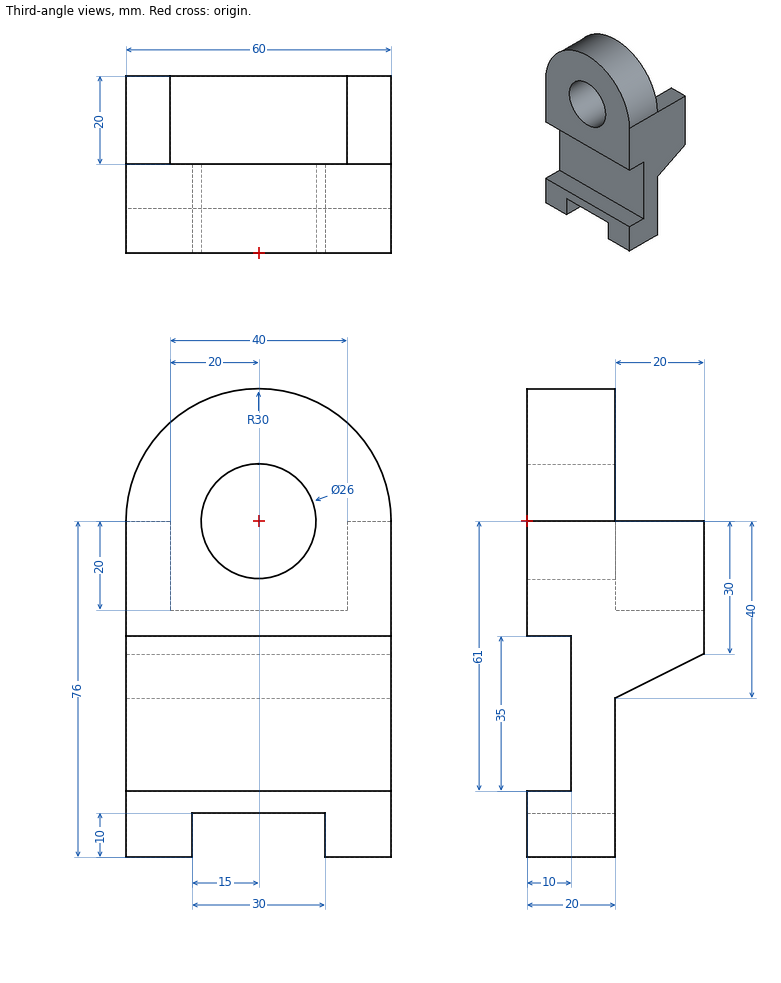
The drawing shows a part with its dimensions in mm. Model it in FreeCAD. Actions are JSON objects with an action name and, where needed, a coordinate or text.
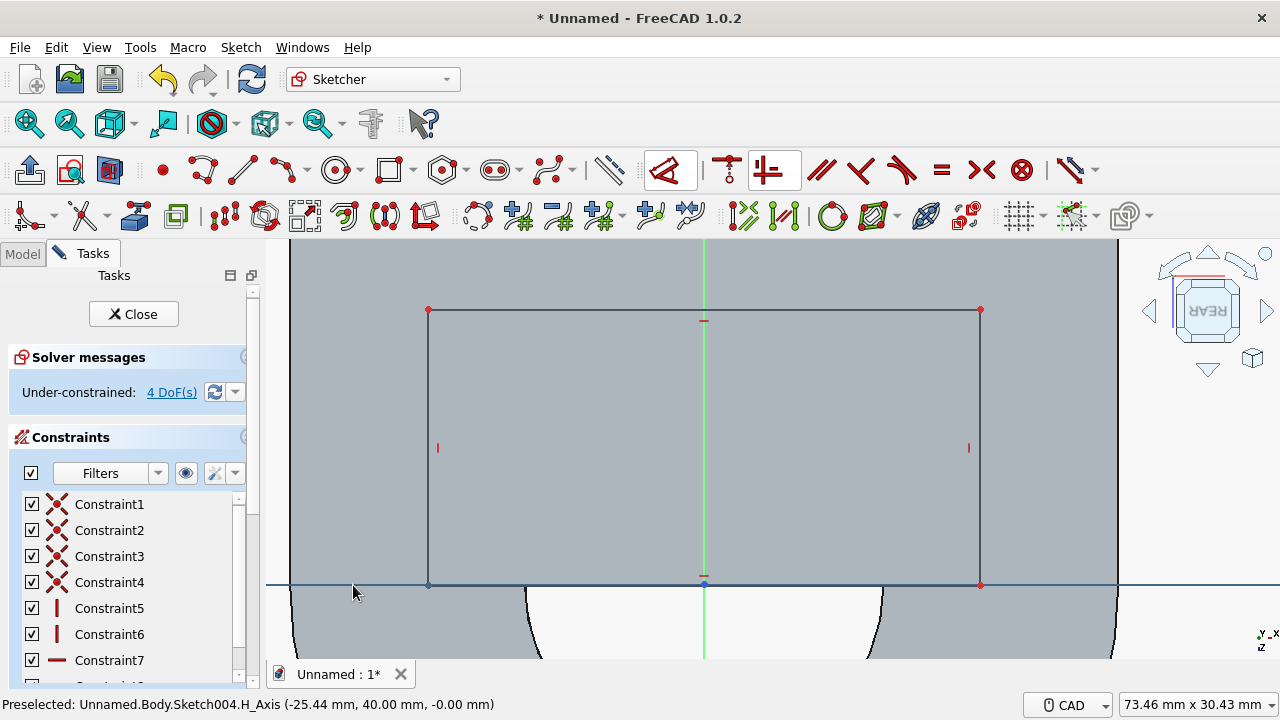
{"action": "key", "text": "c"}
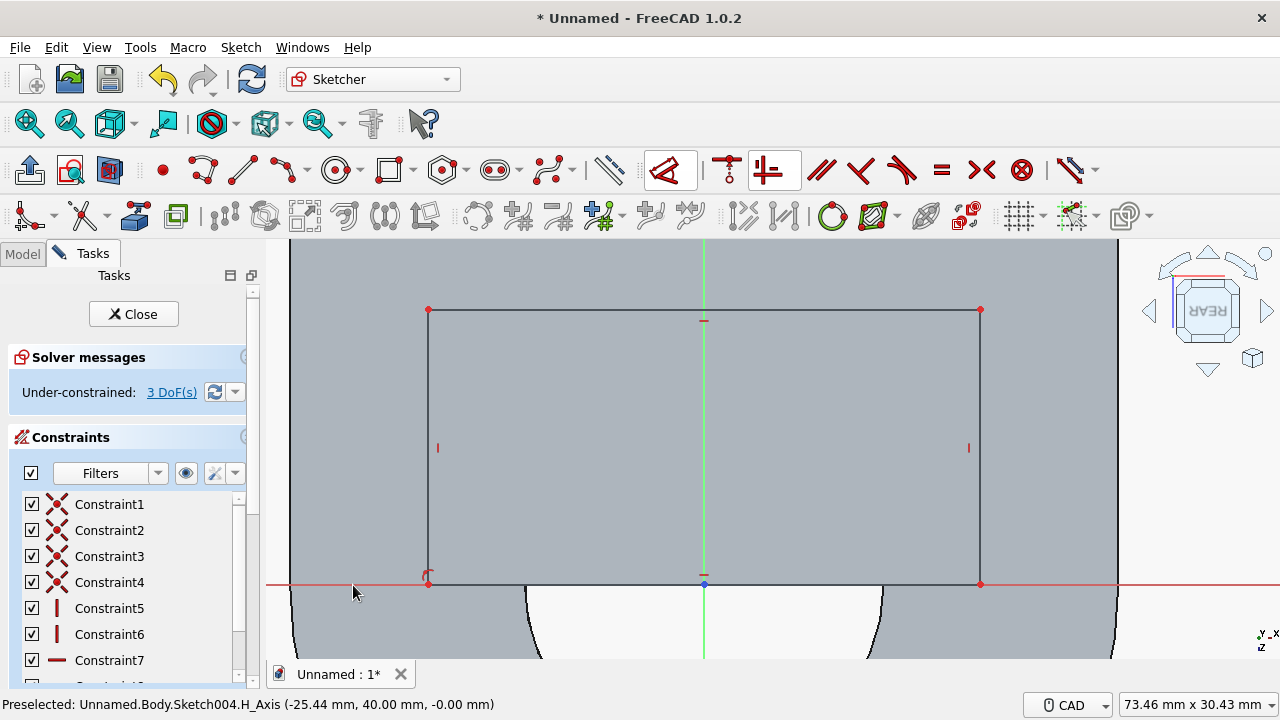
{"action": "left_click", "coordinate": [428, 392]}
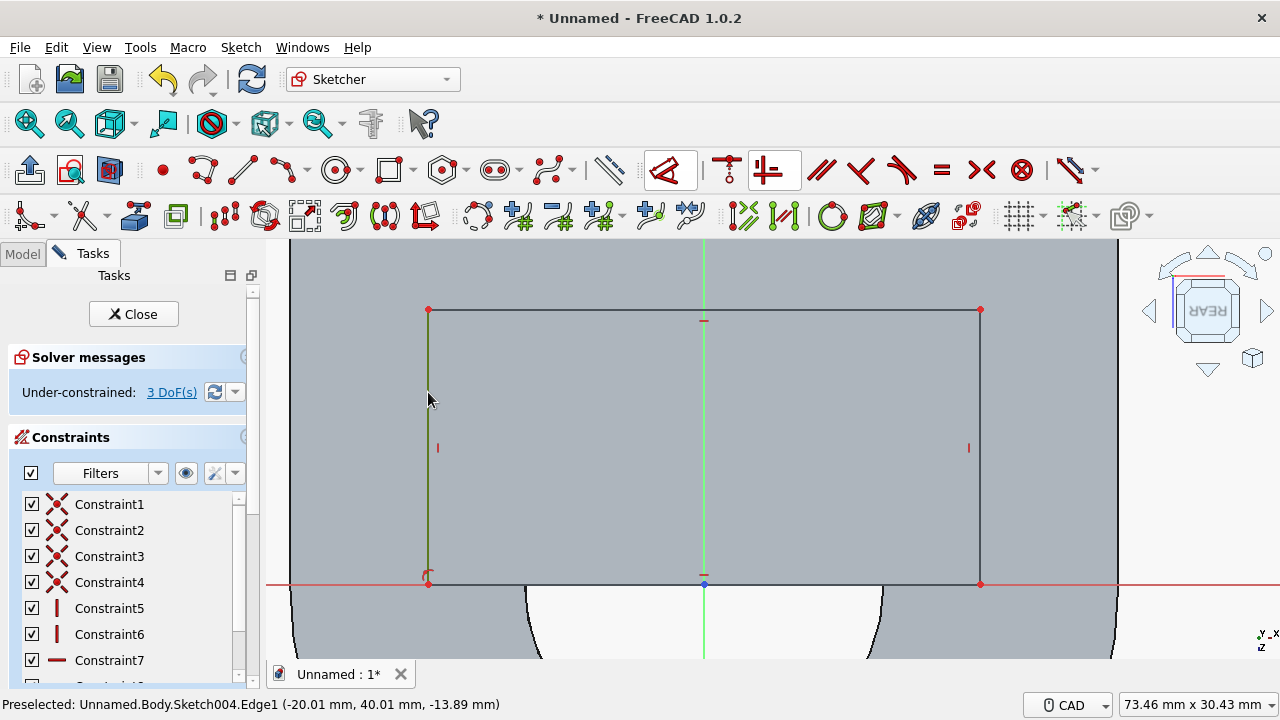
{"action": "left_click", "coordinate": [692, 170]}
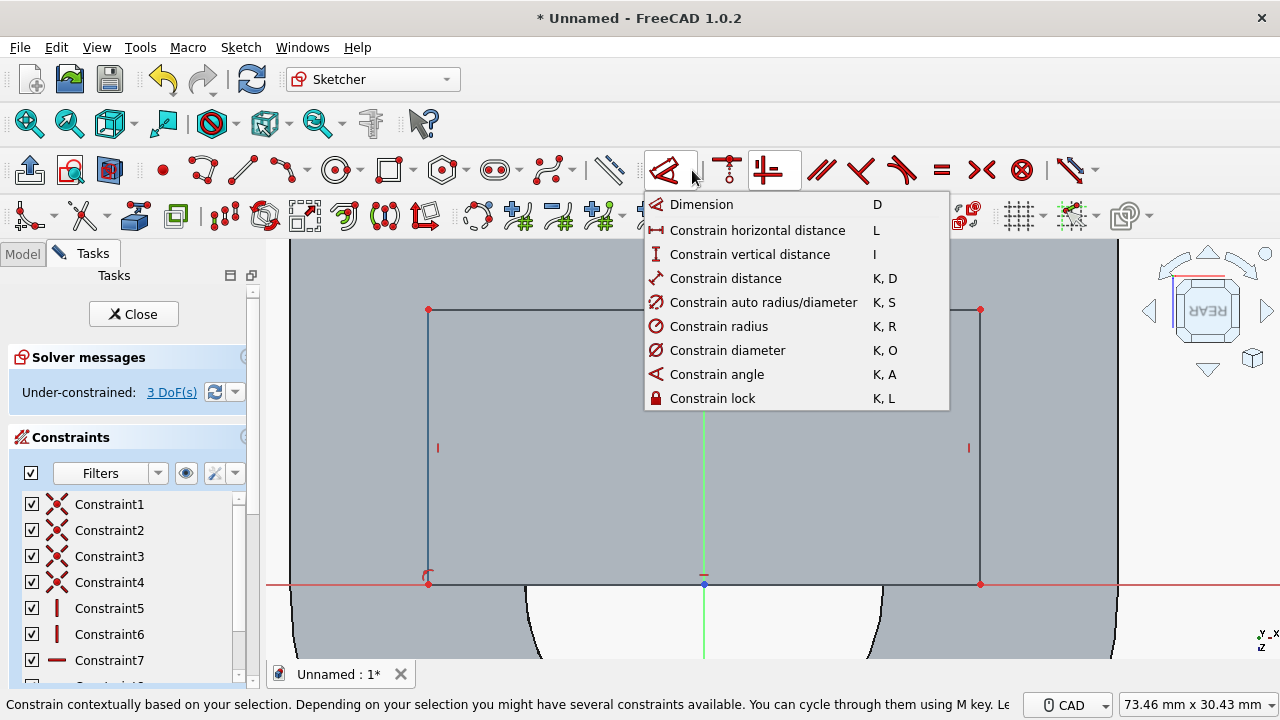
{"action": "left_click", "coordinate": [797, 254]}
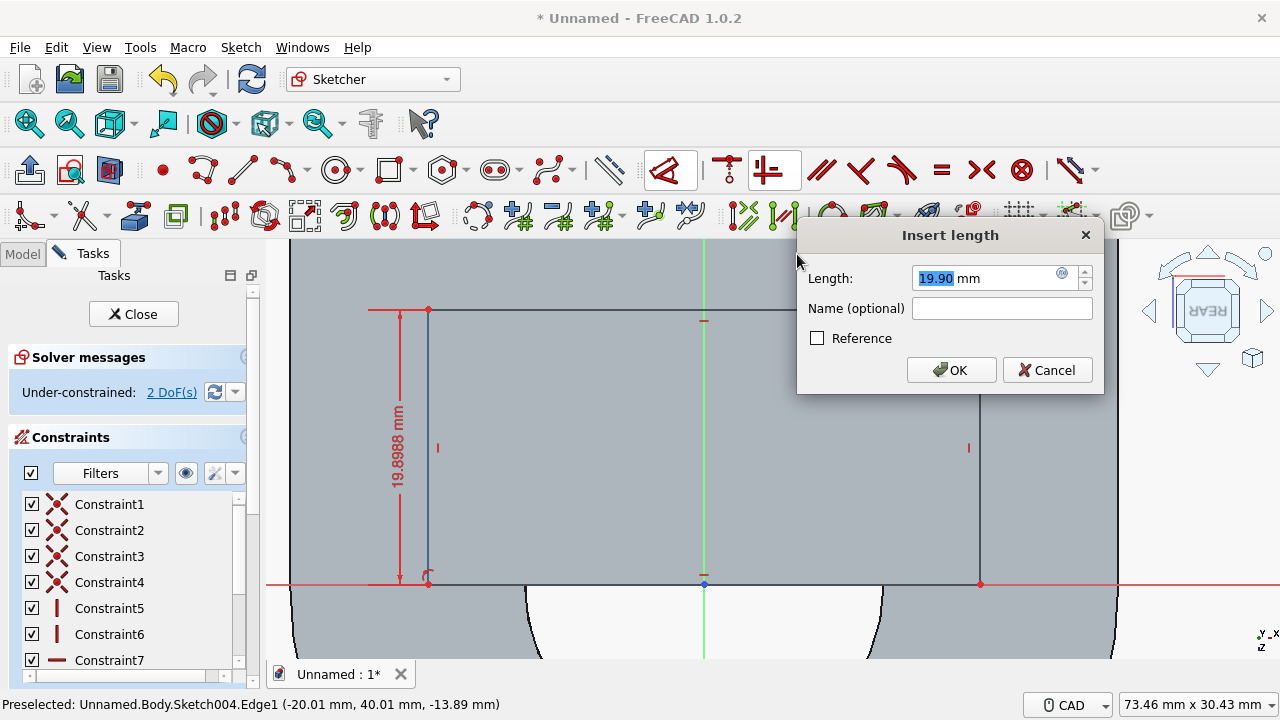
{"action": "type", "text": "20"}
{"action": "key", "text": "Return"}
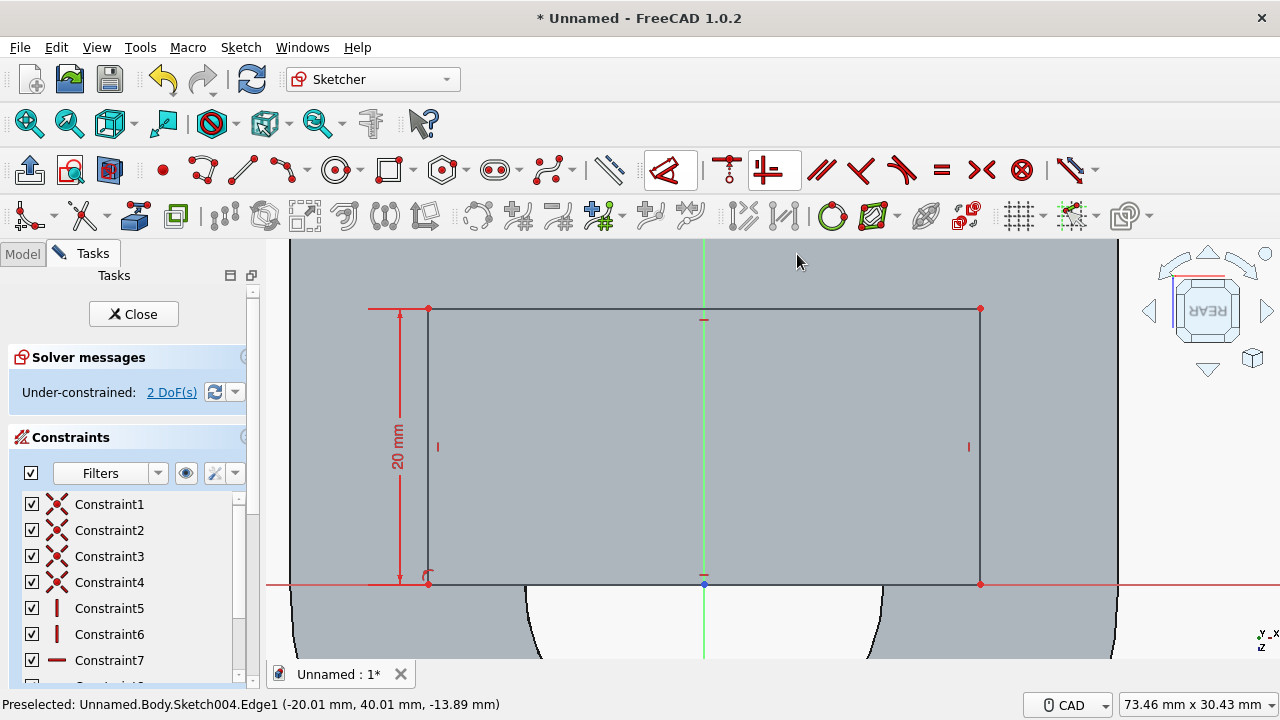
{"action": "left_click", "coordinate": [594, 585]}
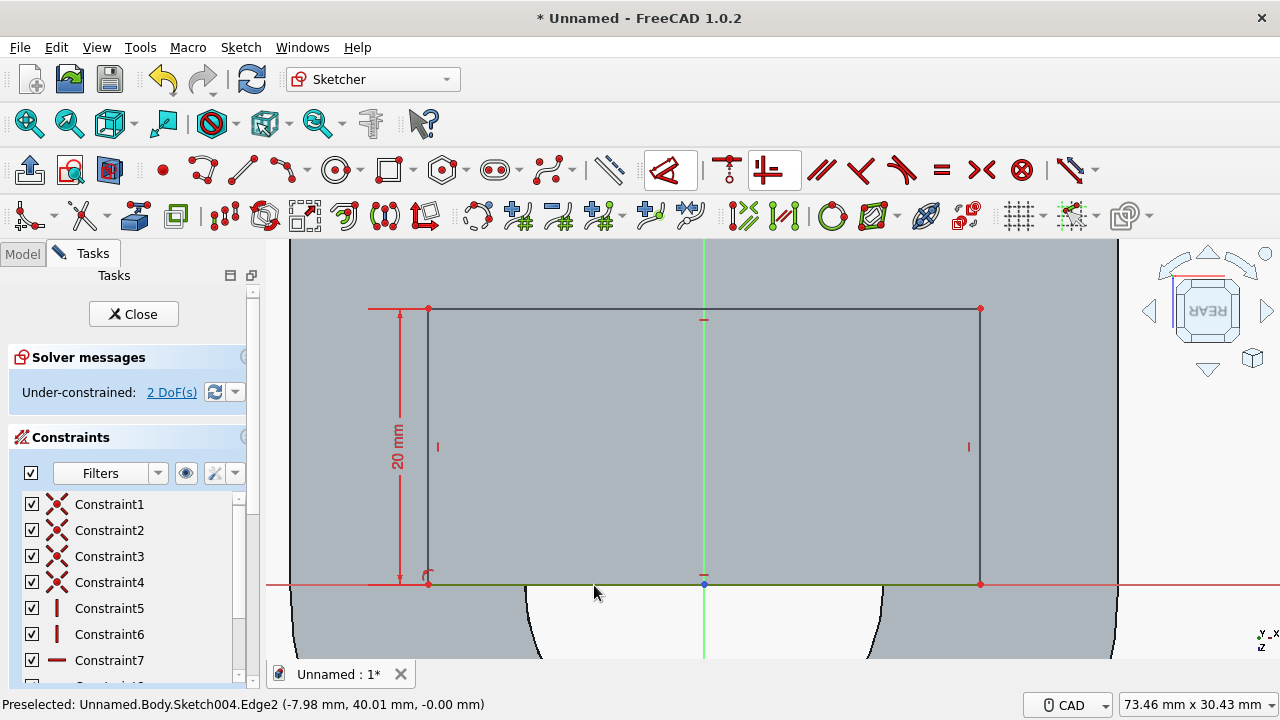
{"action": "key", "text": "l"}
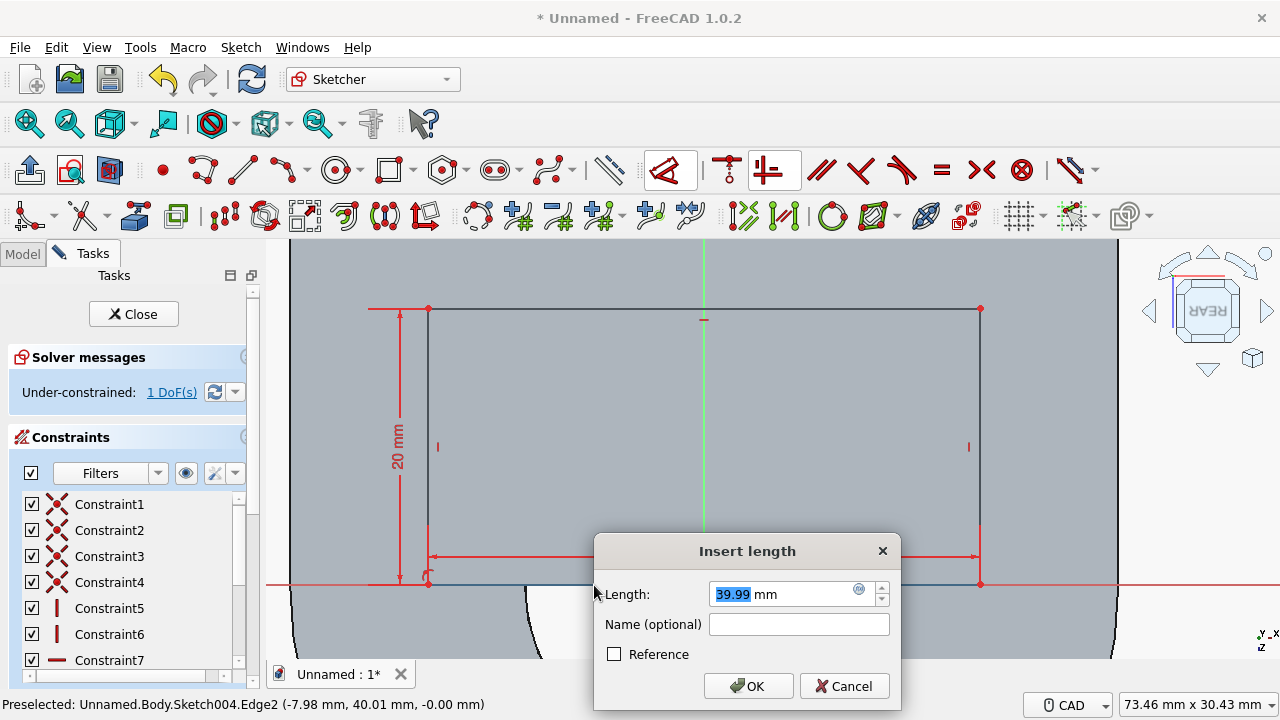
{"action": "type", "text": "40"}
{"action": "key", "text": "Return"}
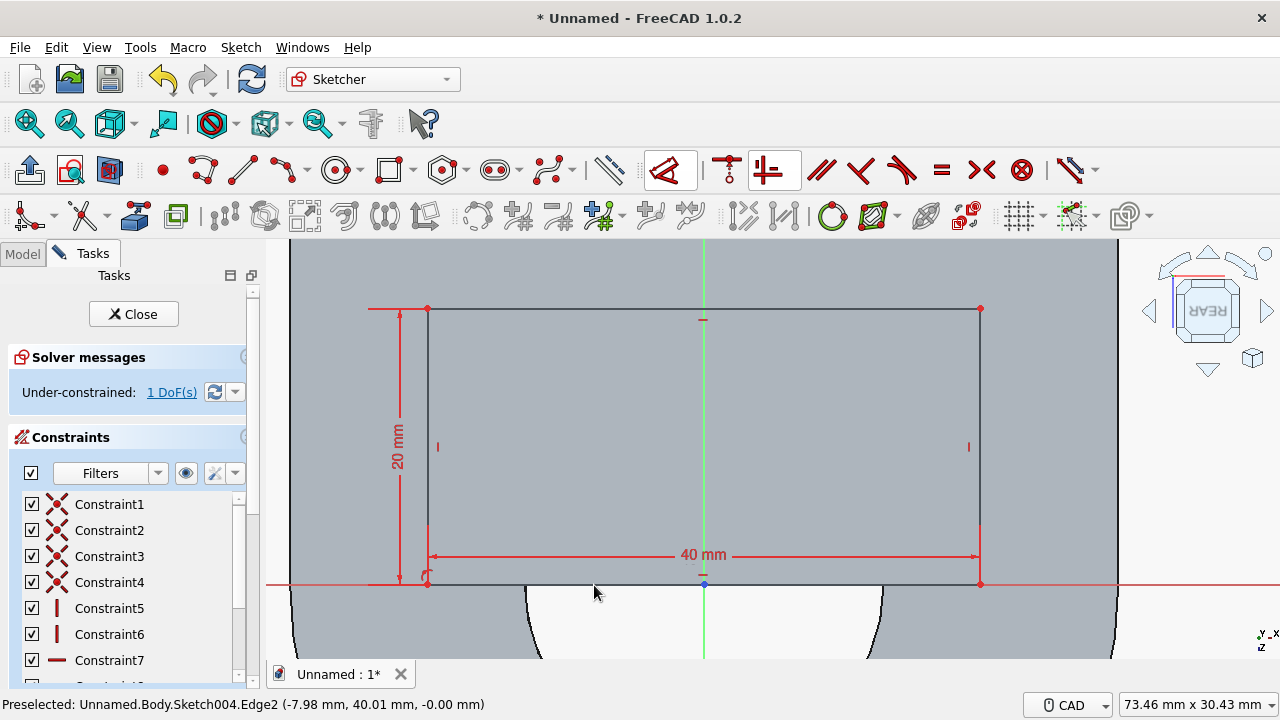
{"action": "left_click", "coordinate": [428, 309]}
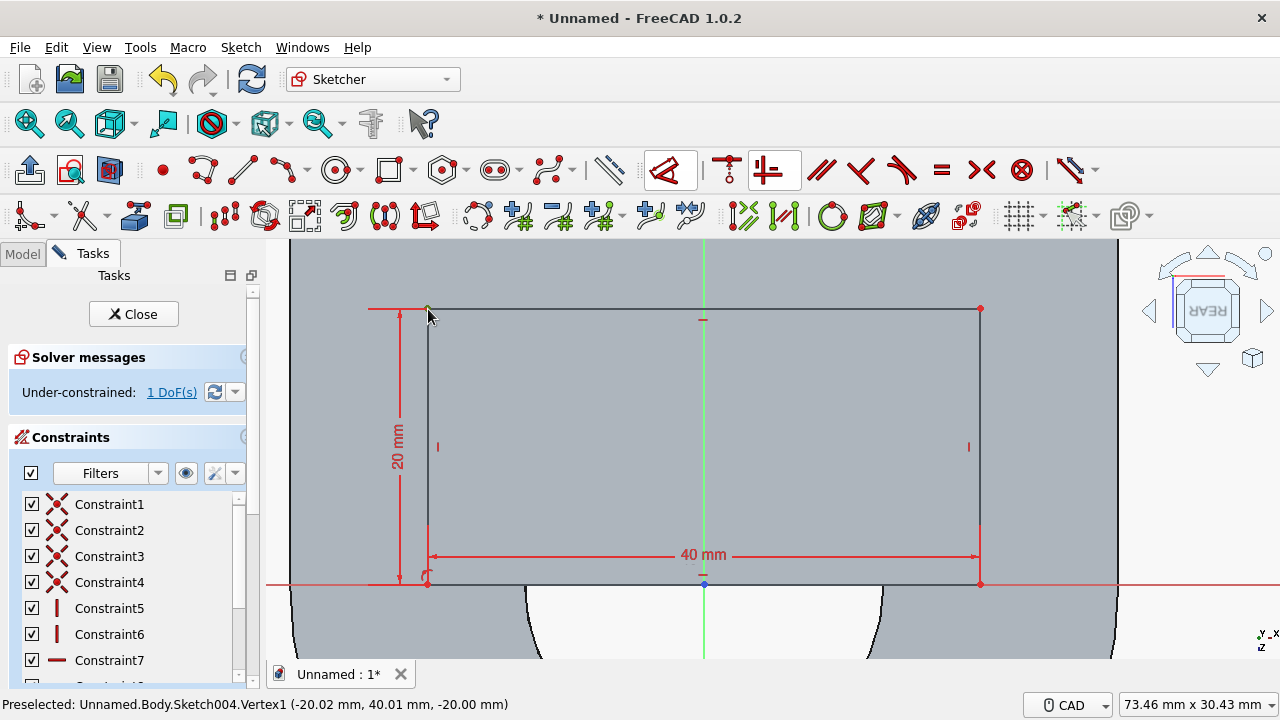
{"action": "key", "text": "l"}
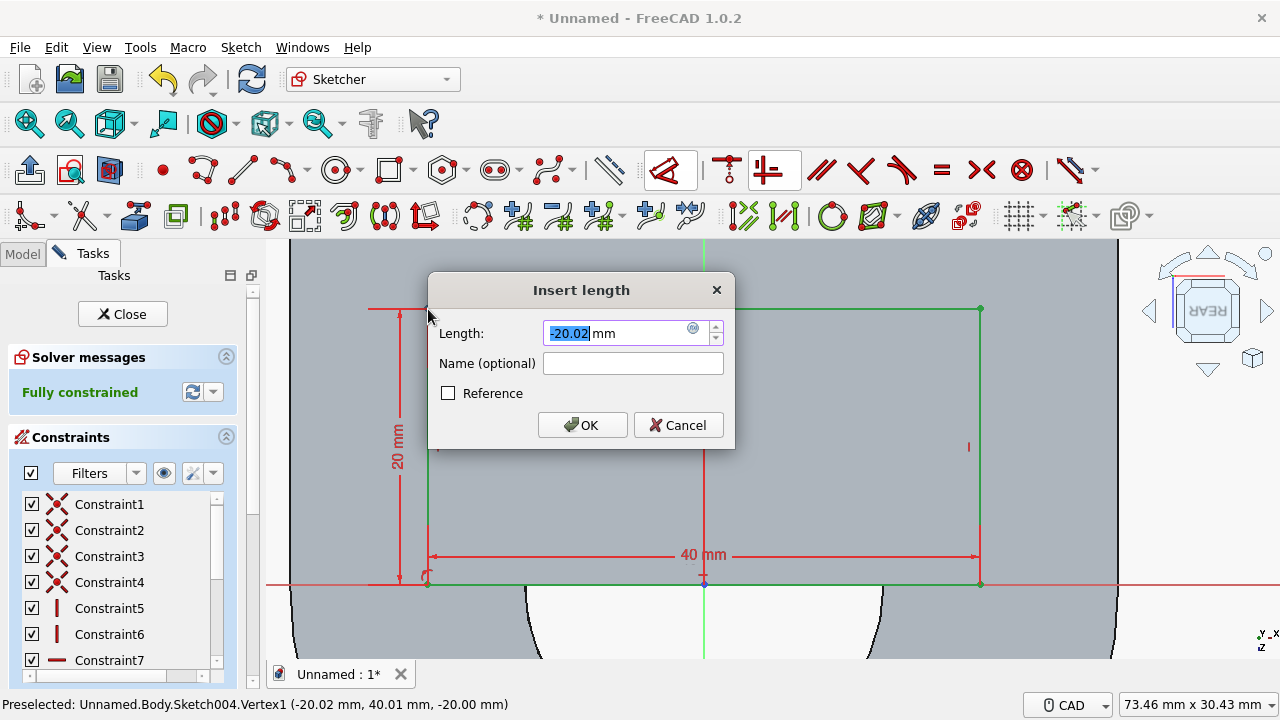
{"action": "type", "text": "-20"}
{"action": "key", "text": "Return"}